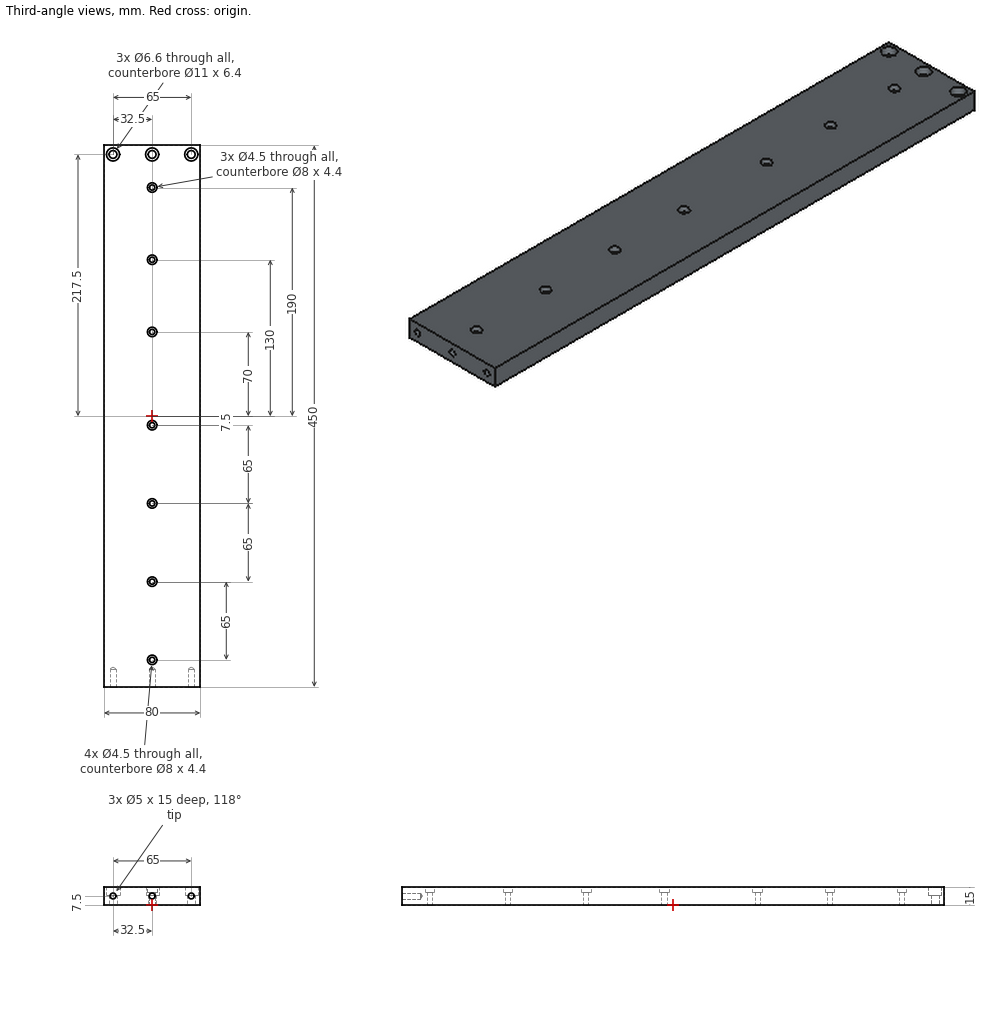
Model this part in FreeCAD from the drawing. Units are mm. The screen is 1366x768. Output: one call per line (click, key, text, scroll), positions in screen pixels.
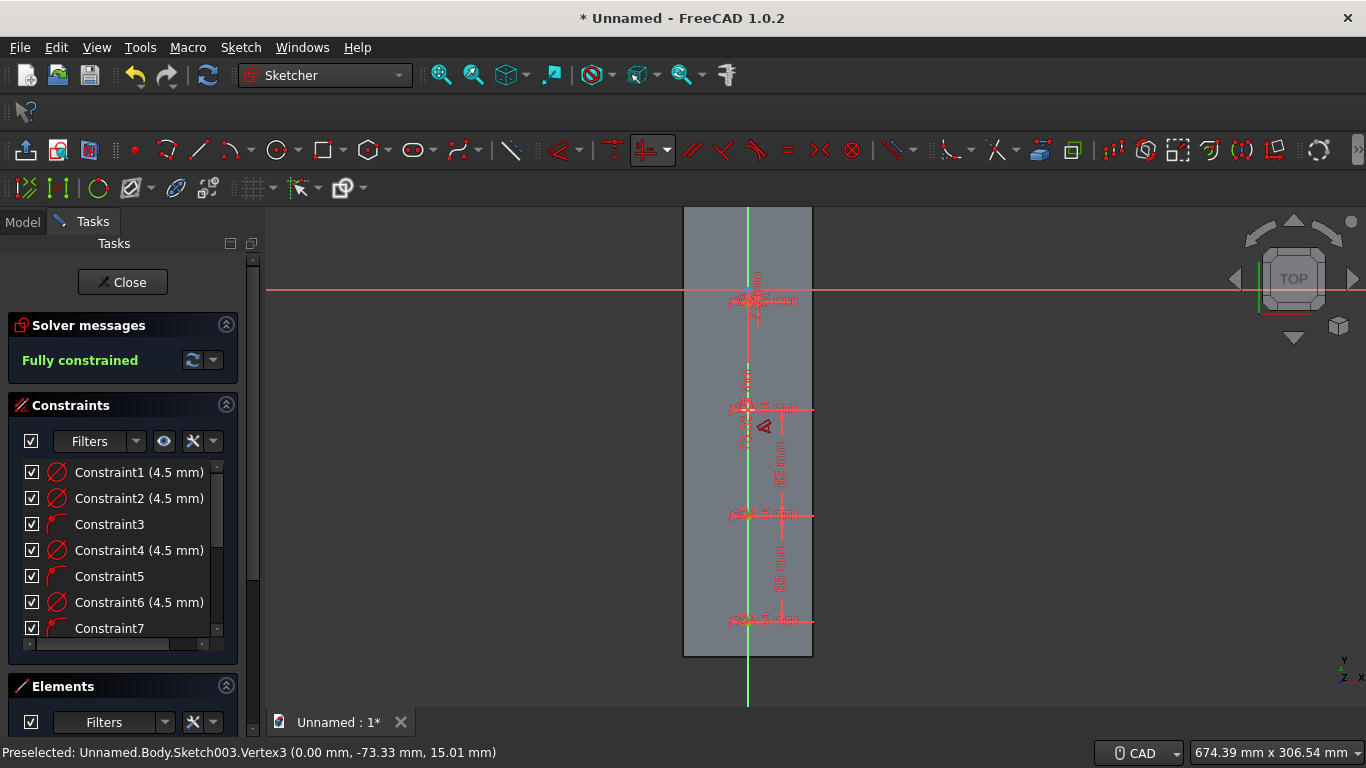
click(748, 302)
click(782, 356)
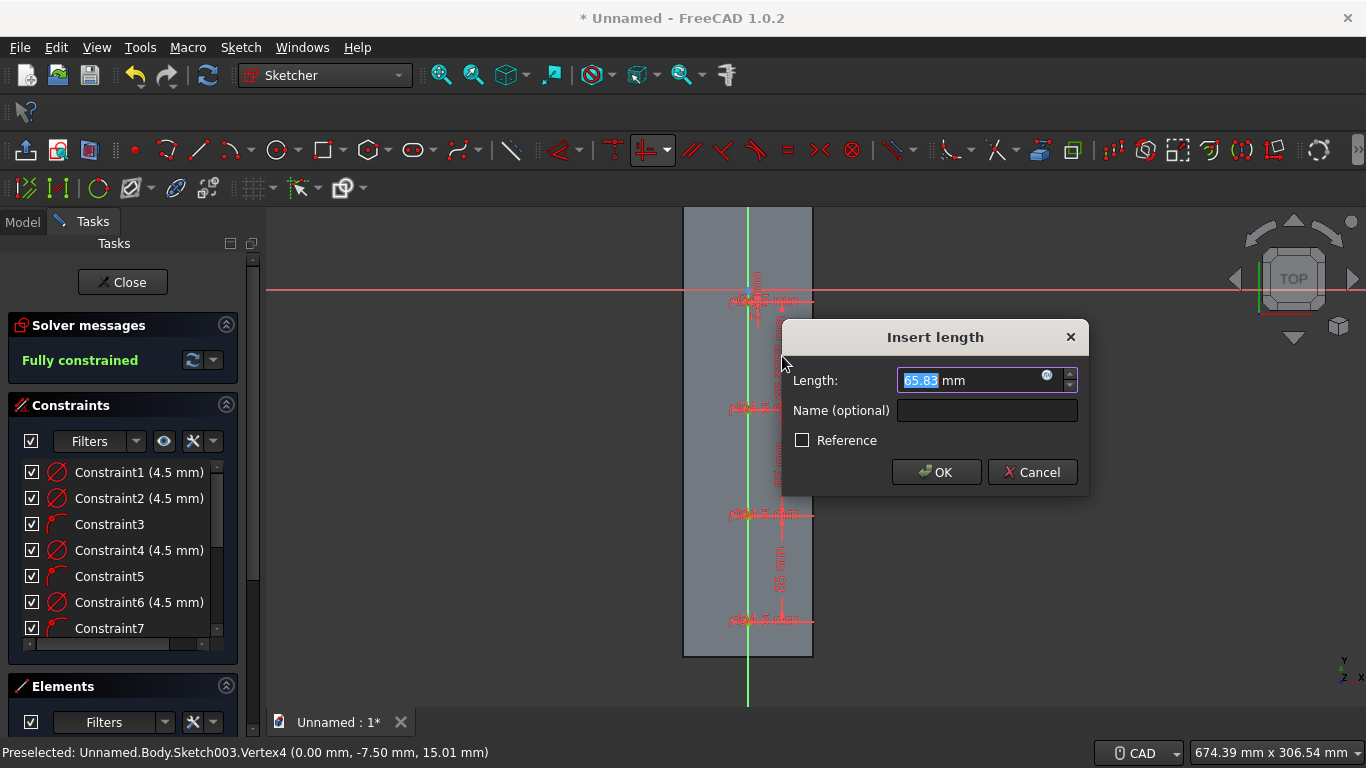
text(65)
key(Return)
key(Escape)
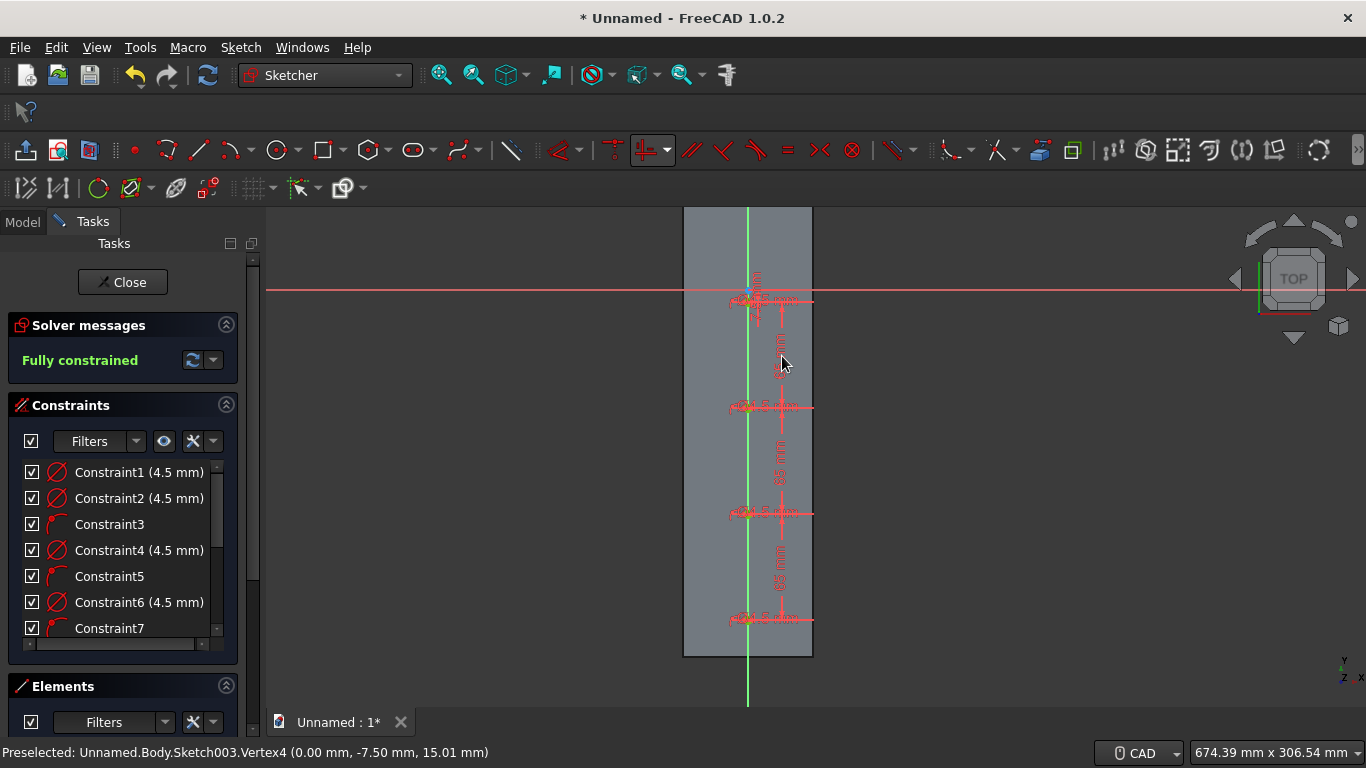
click(123, 282)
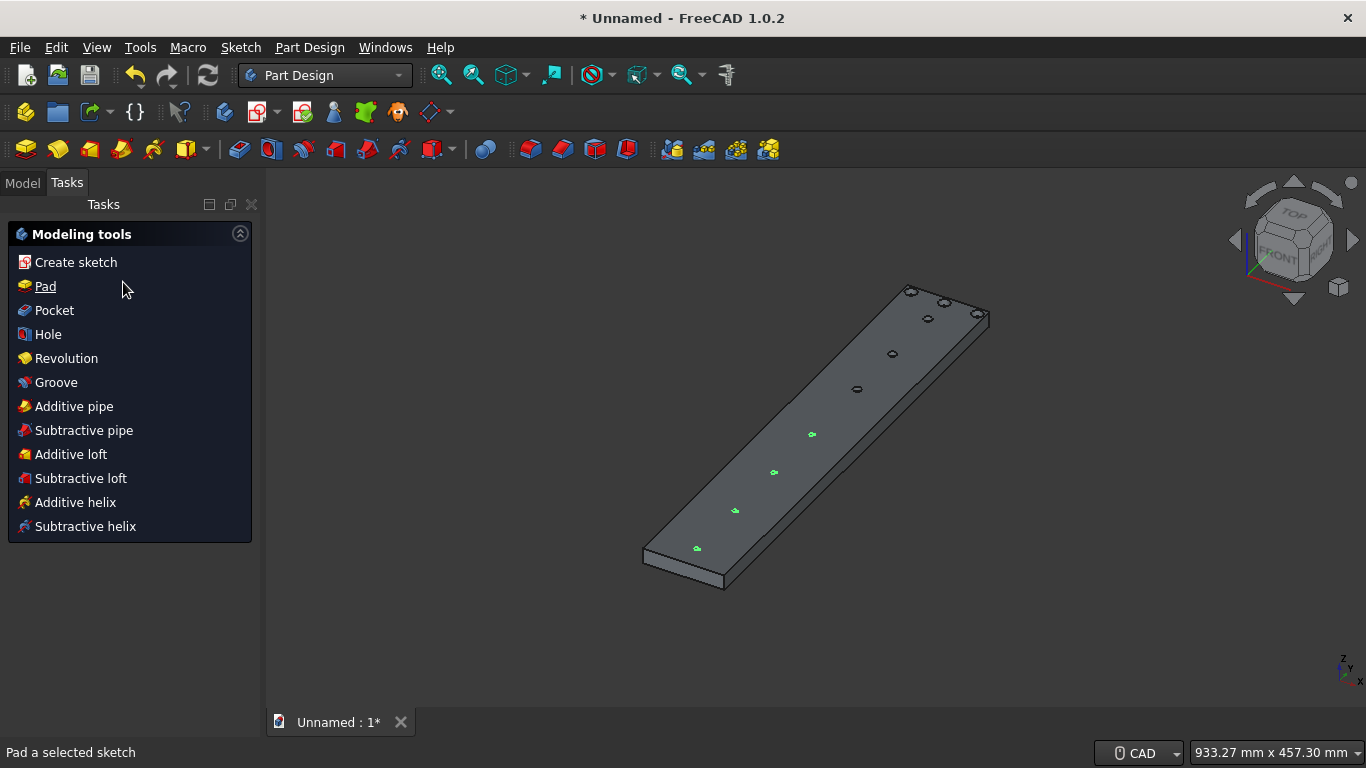
click(272, 150)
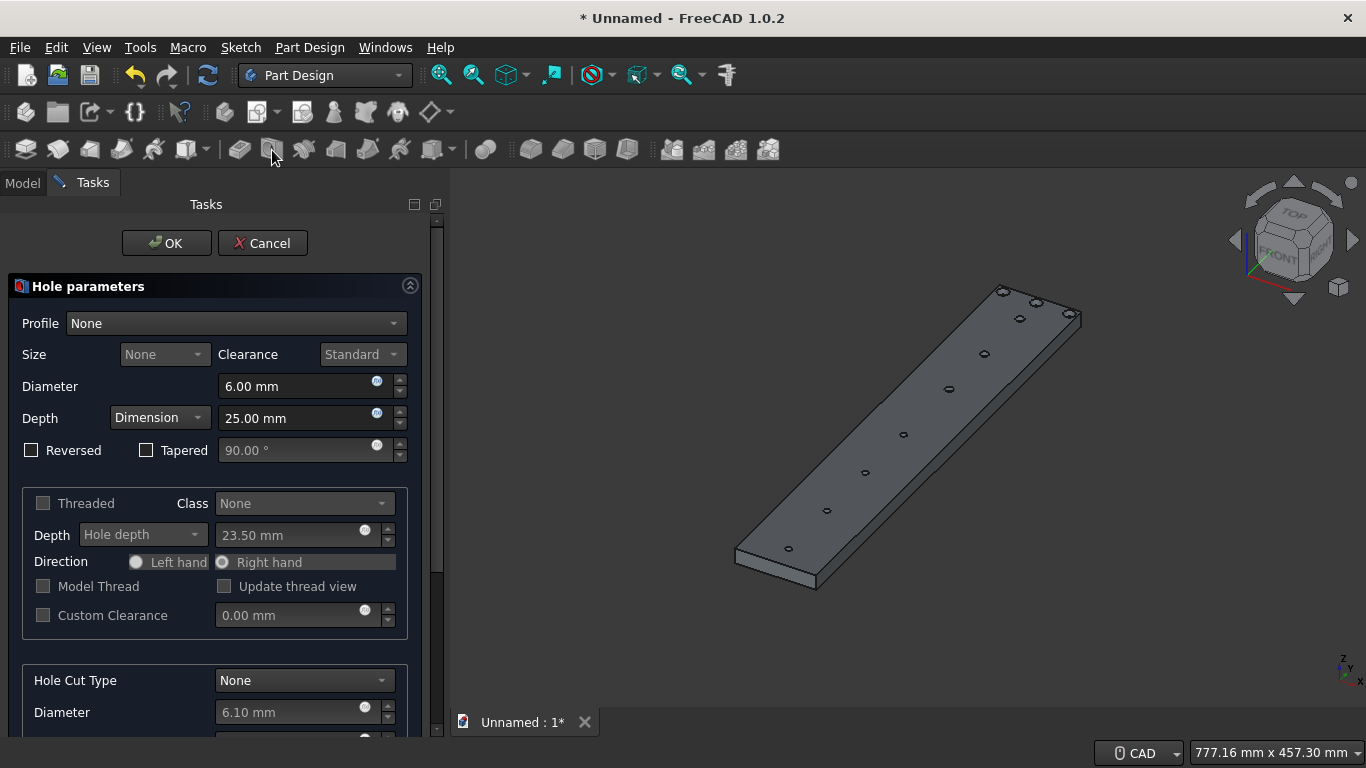
triple_click(305, 386)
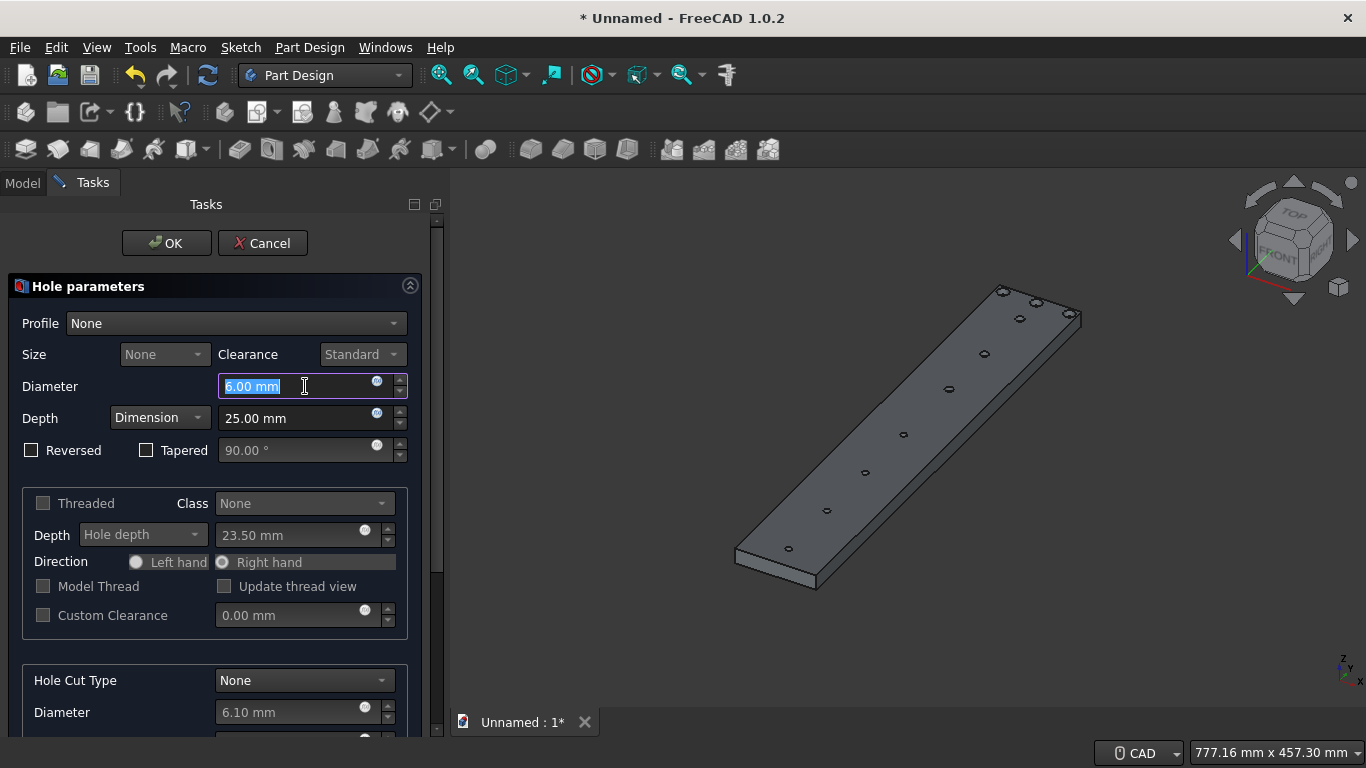
text(4.5)
key(Tab)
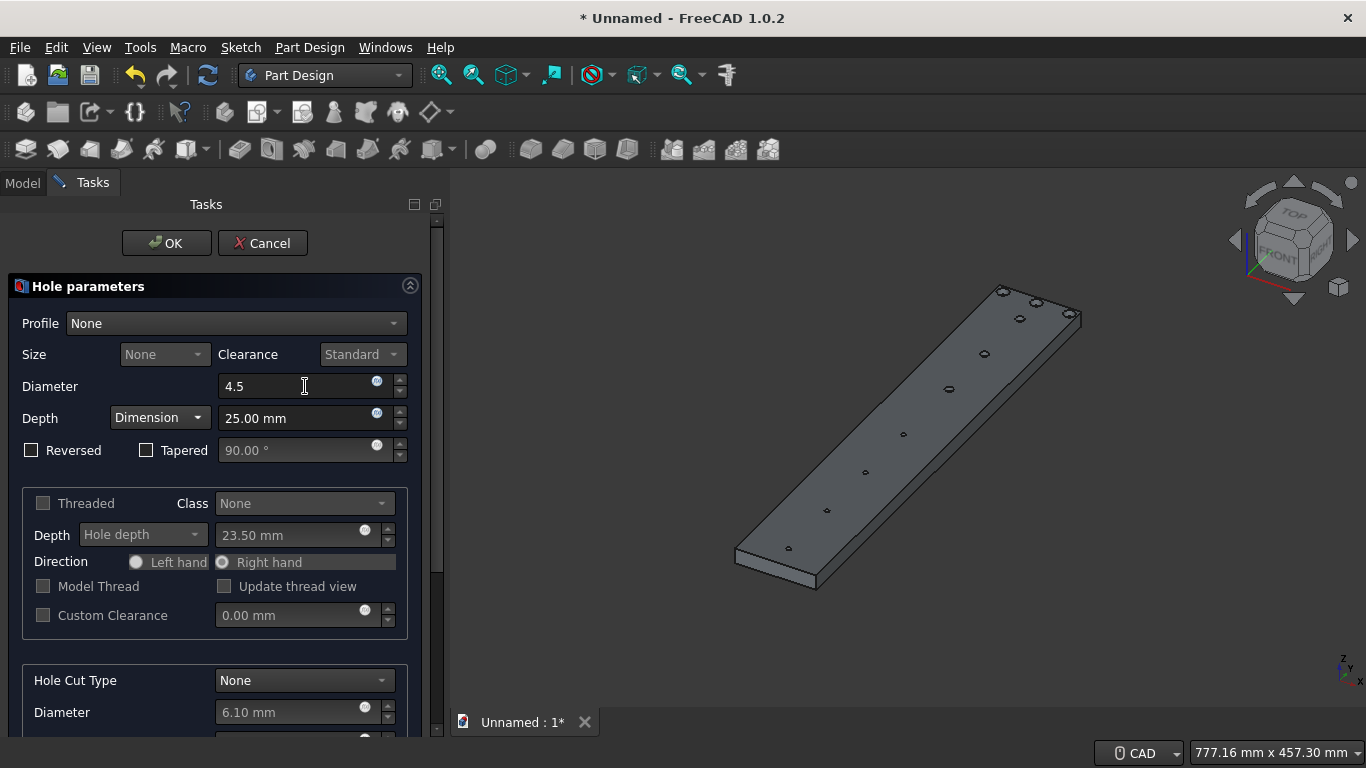
click(161, 418)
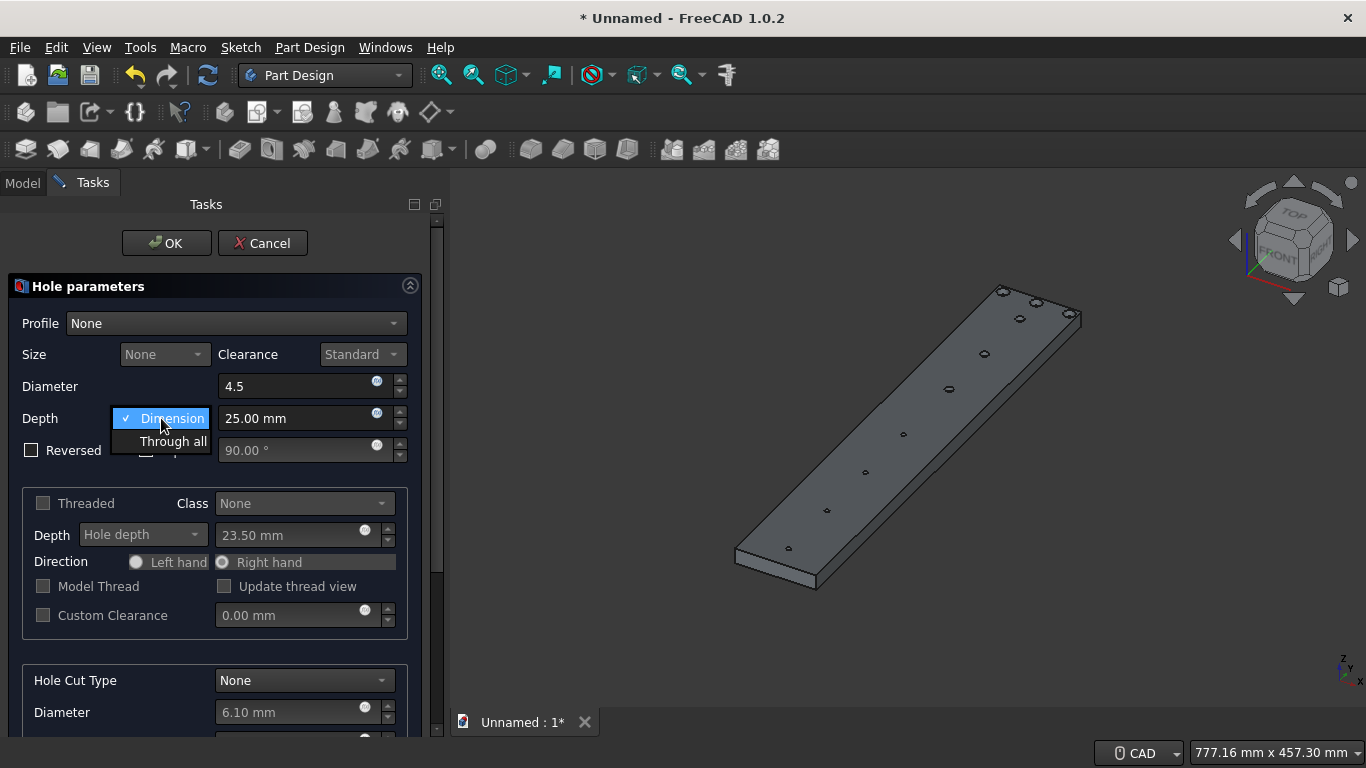
click(160, 442)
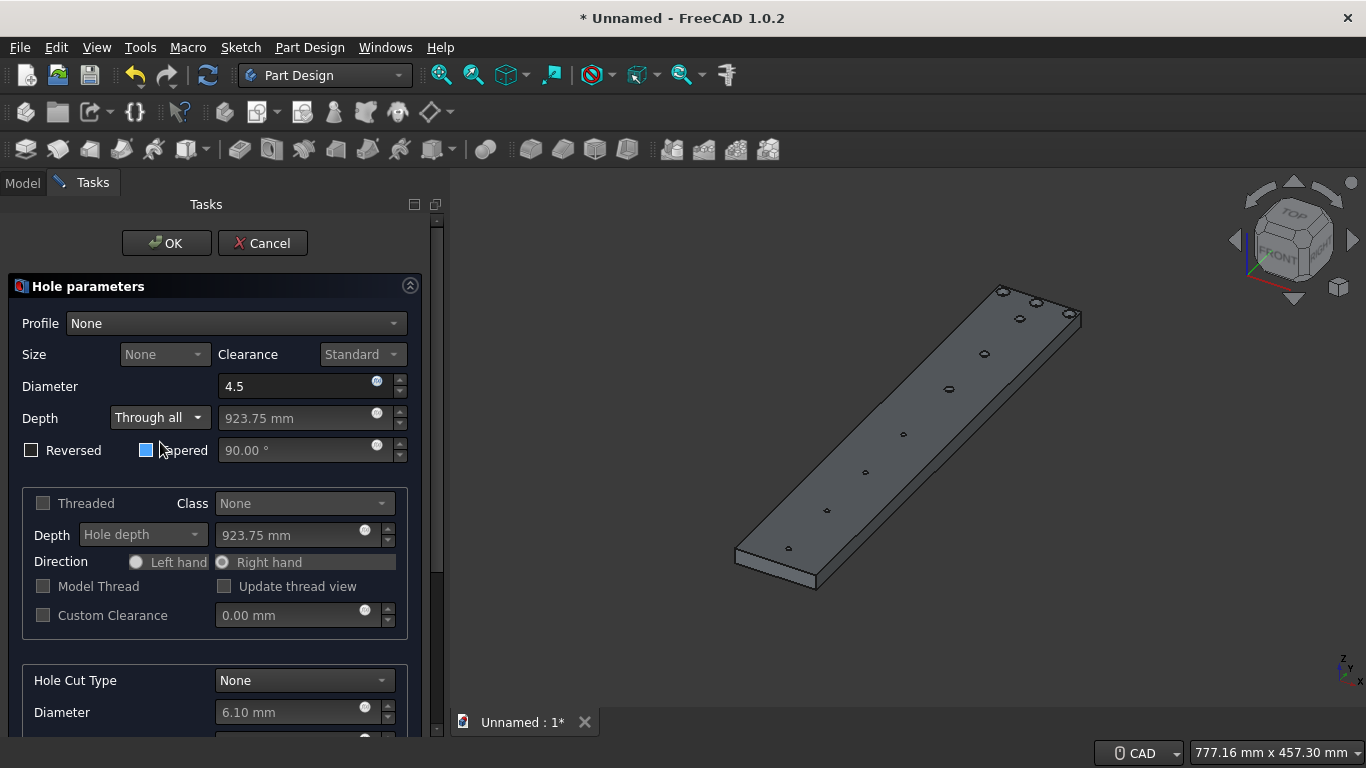
click(306, 680)